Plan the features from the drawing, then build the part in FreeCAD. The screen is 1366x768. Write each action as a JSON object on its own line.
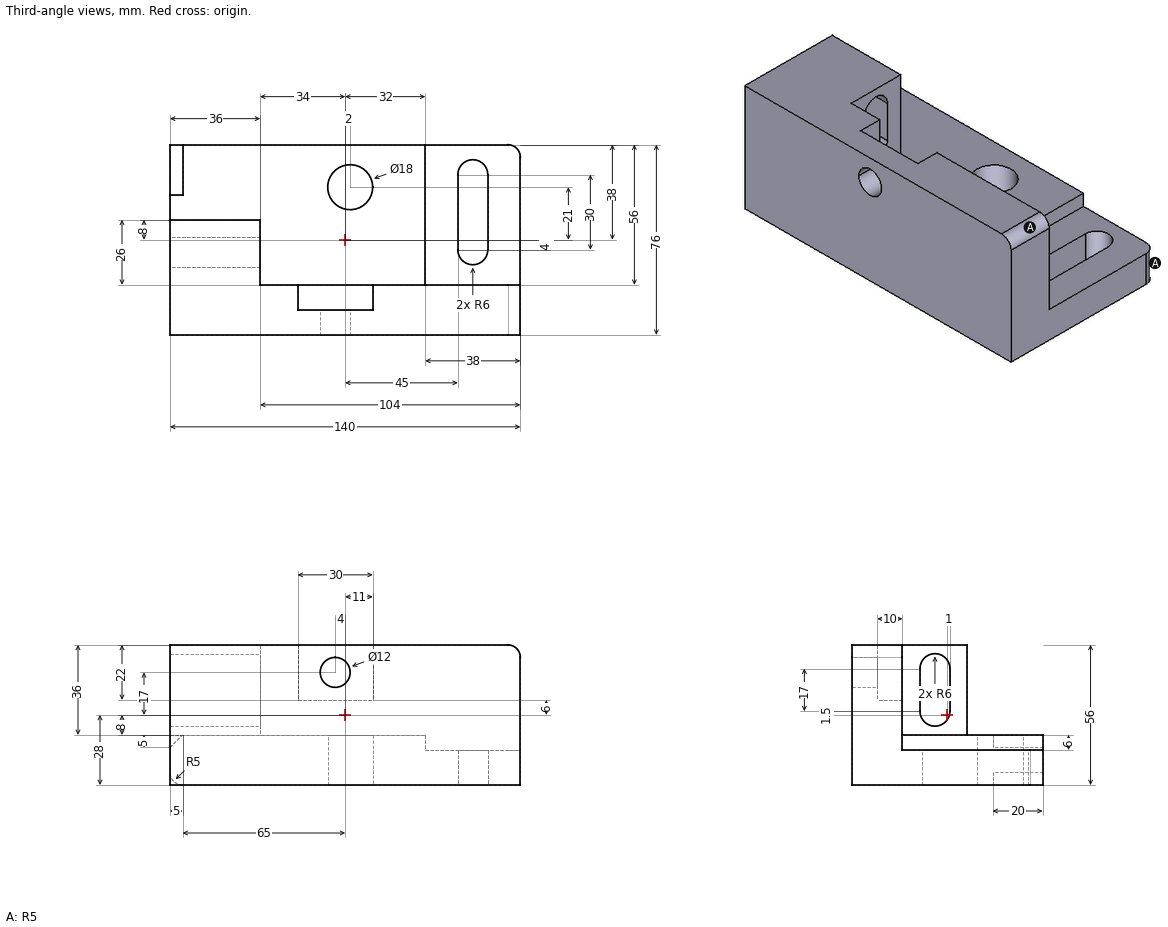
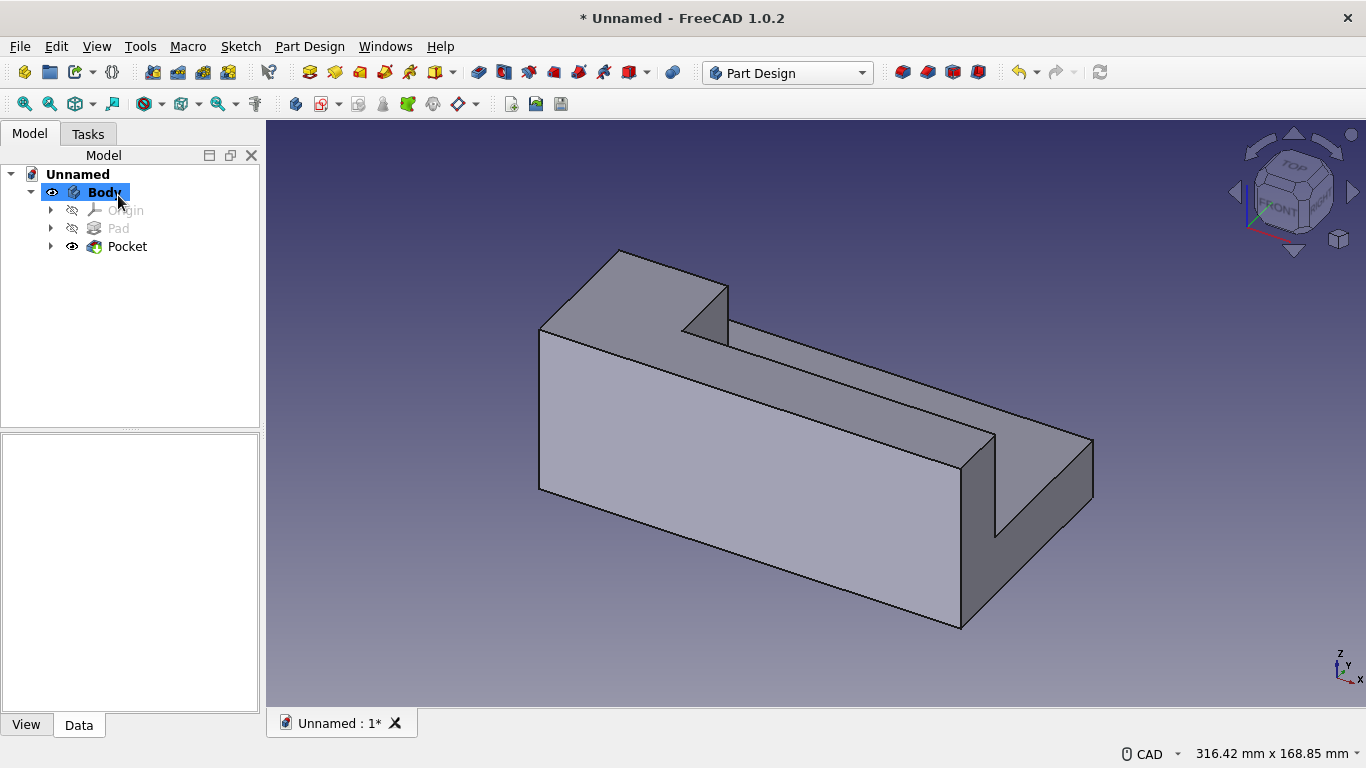
{"action": "key", "text": "4"}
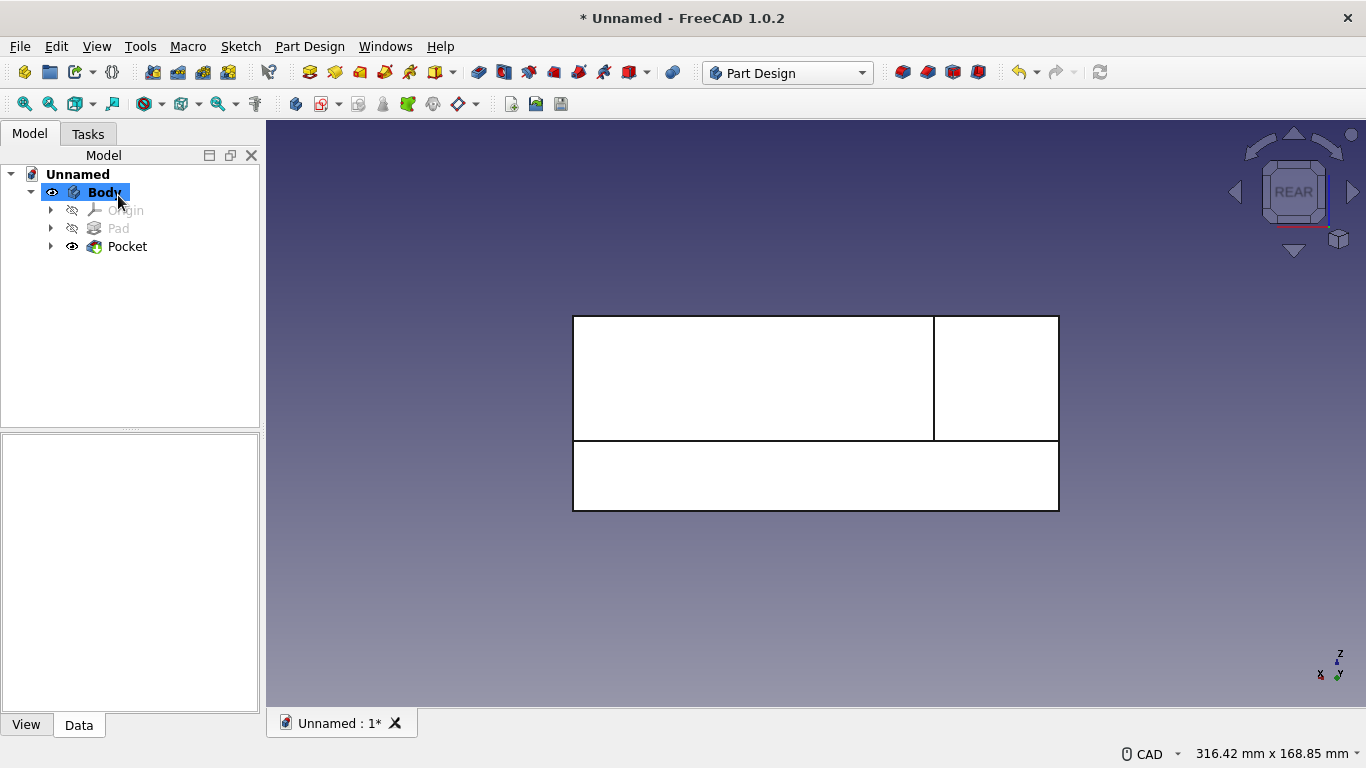
{"action": "key", "text": "v f"}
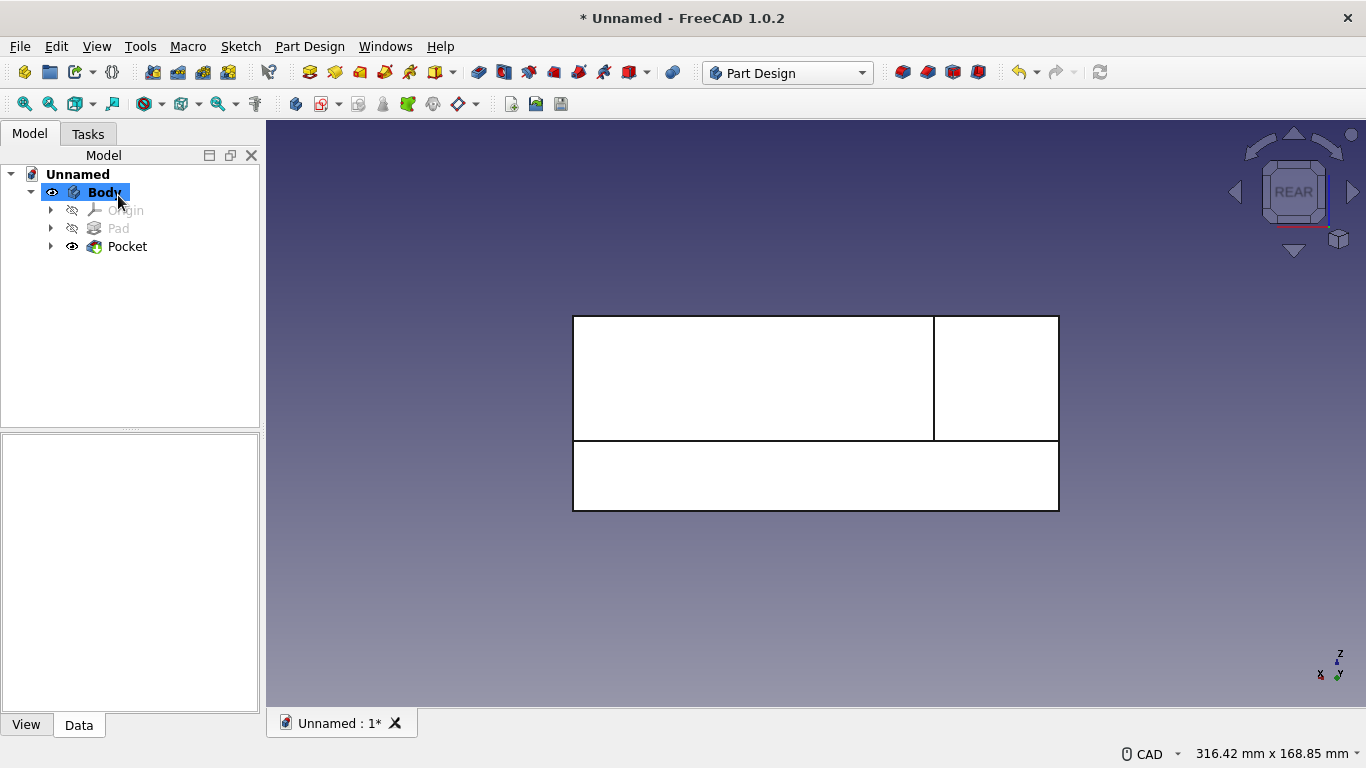
{"action": "left_click", "coordinate": [650, 378]}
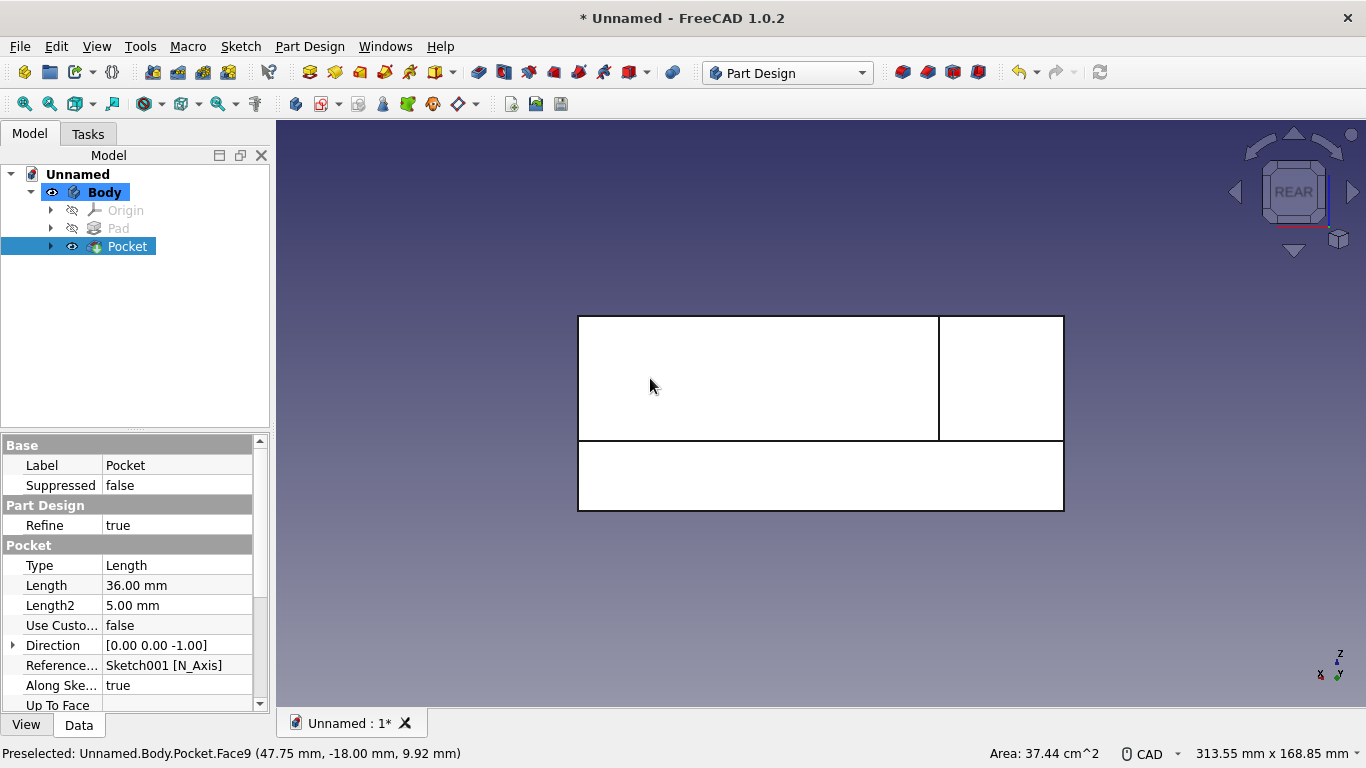
{"action": "left_click", "coordinate": [320, 104]}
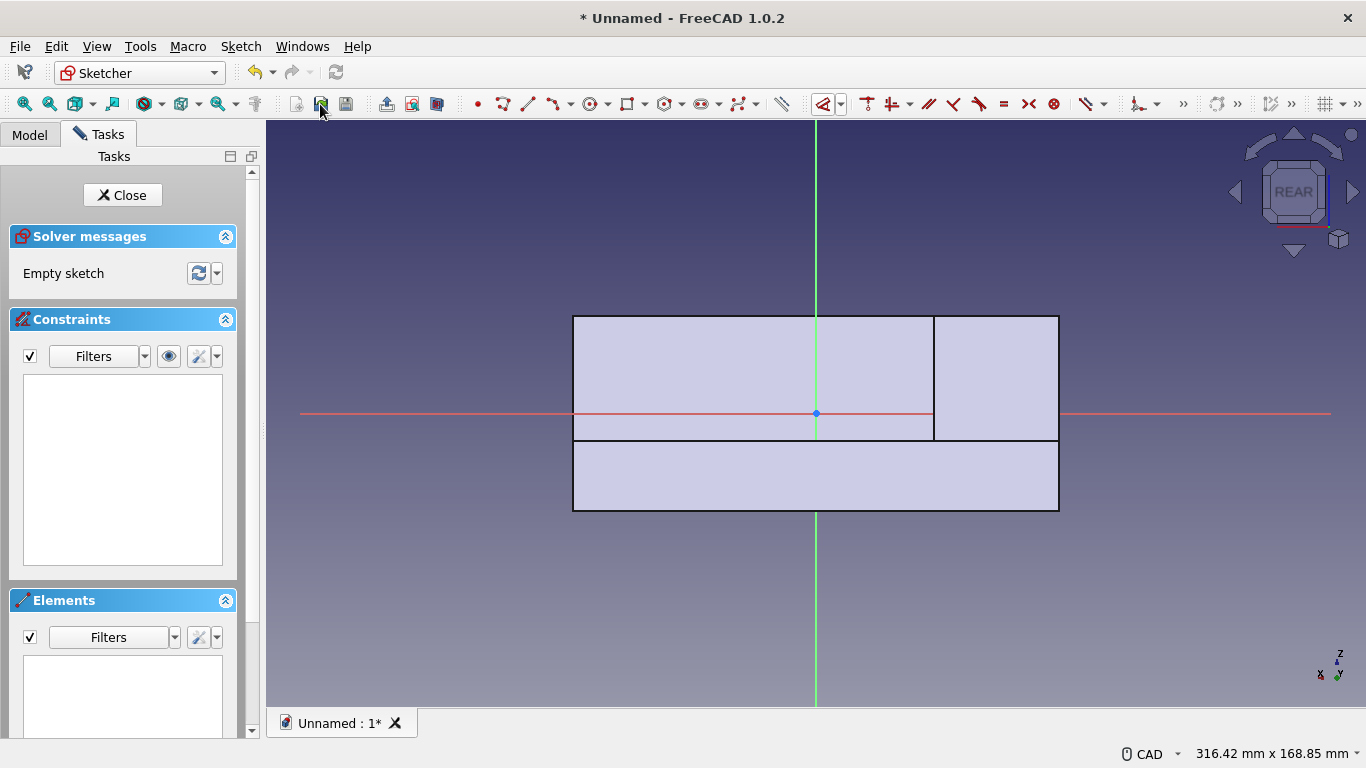
{"action": "scroll", "coordinate": [857, 349], "scroll_direction": "up", "scroll_amount": 7}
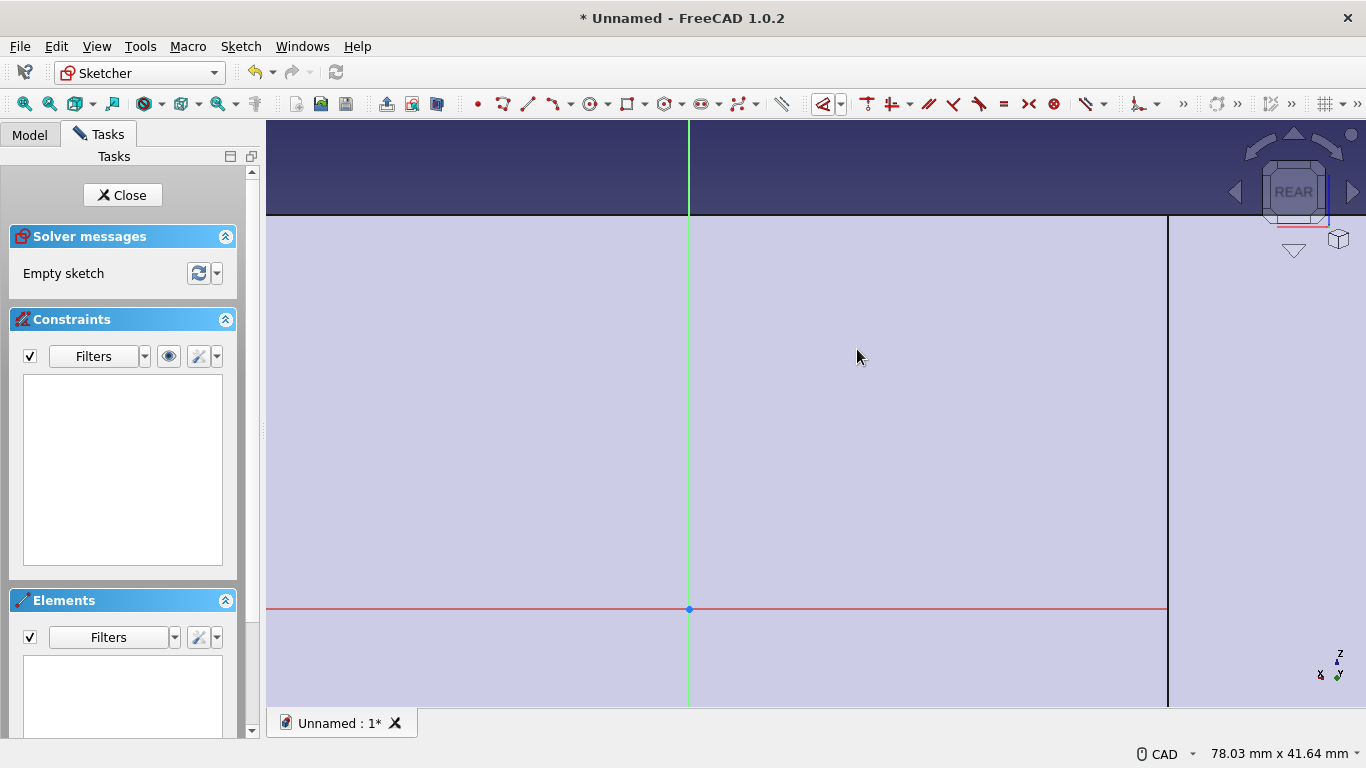
{"action": "left_click", "coordinate": [626, 104]}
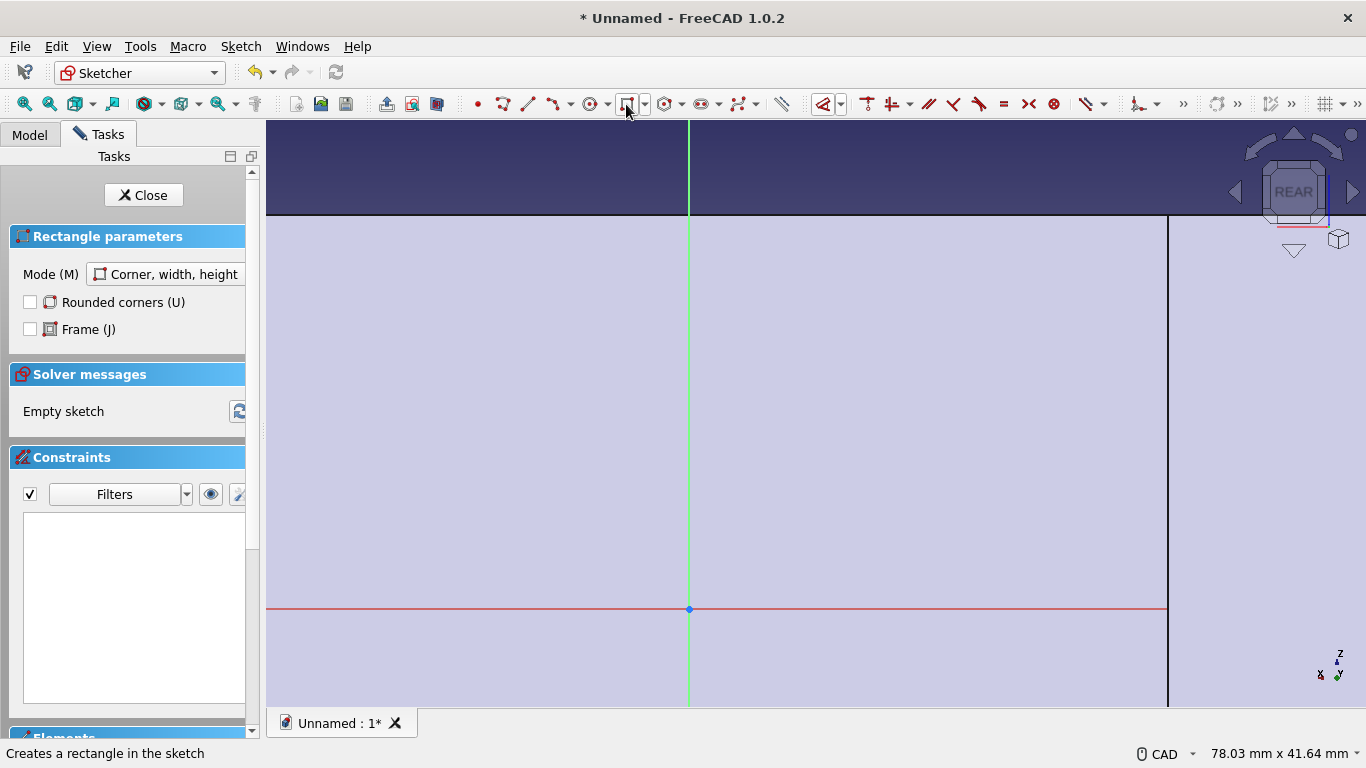
{"action": "left_click", "coordinate": [534, 215]}
{"action": "mouse_move", "coordinate": [957, 525]}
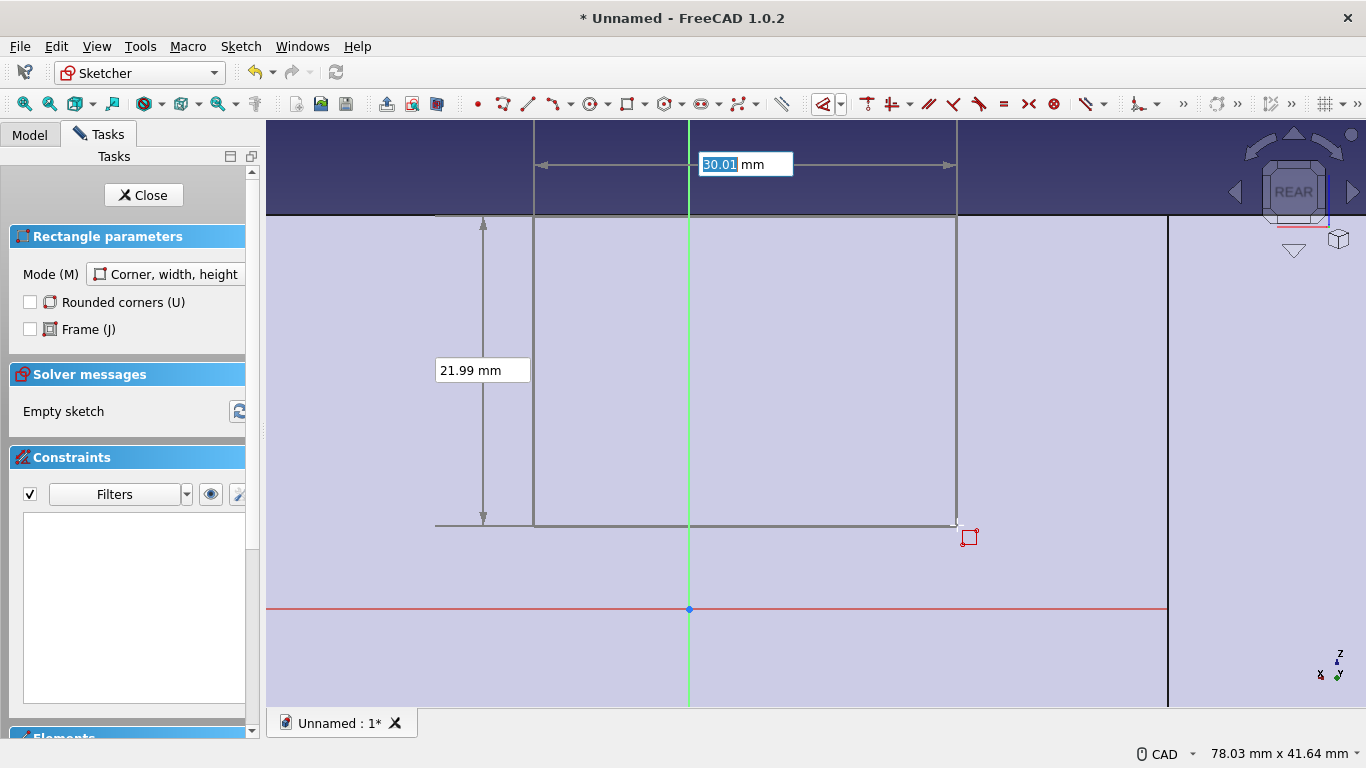
{"action": "type", "text": "30"}
{"action": "key", "text": "Tab"}
{"action": "type", "text": "22"}
{"action": "key", "text": "Return"}
{"action": "key", "text": "Escape"}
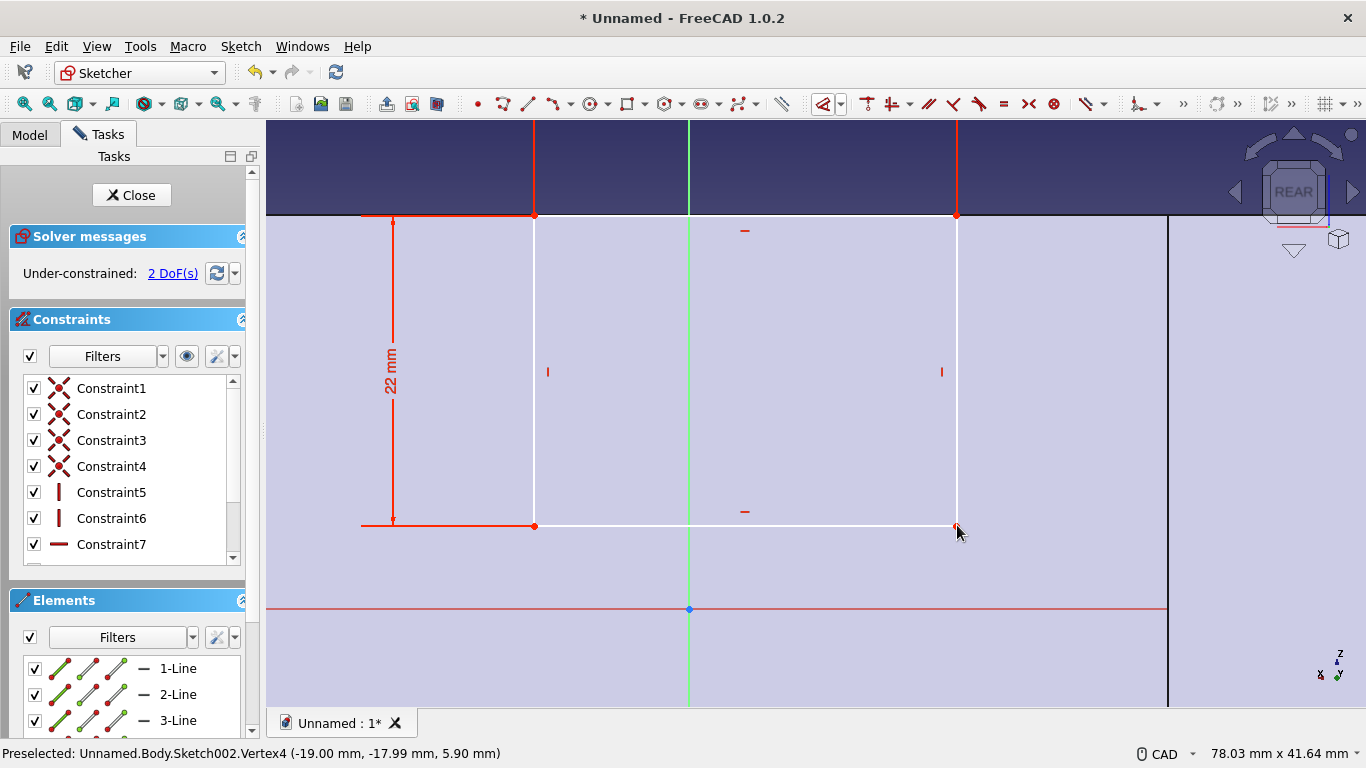
{"action": "left_click", "coordinate": [534, 526]}